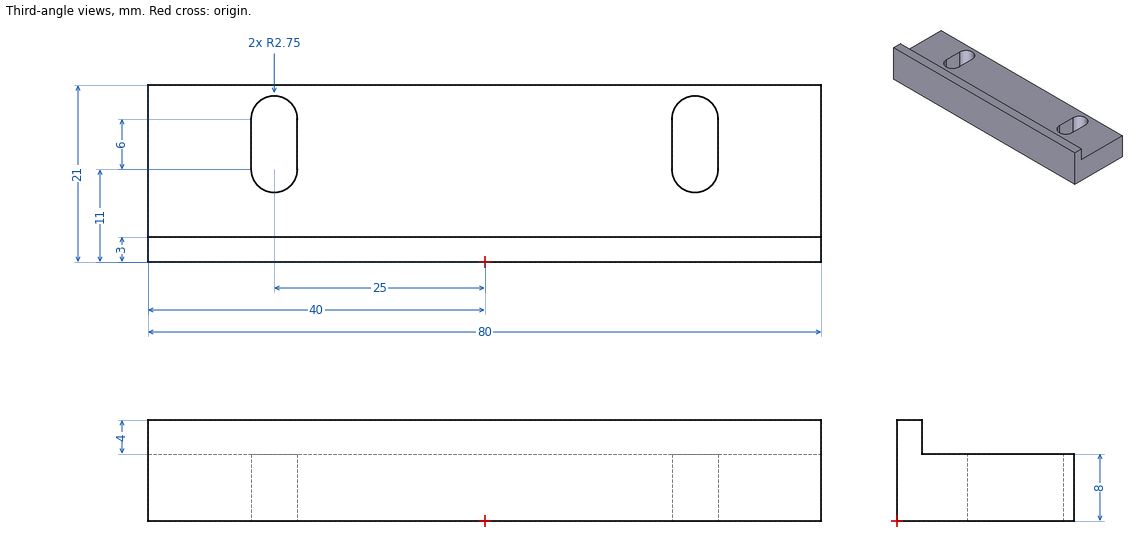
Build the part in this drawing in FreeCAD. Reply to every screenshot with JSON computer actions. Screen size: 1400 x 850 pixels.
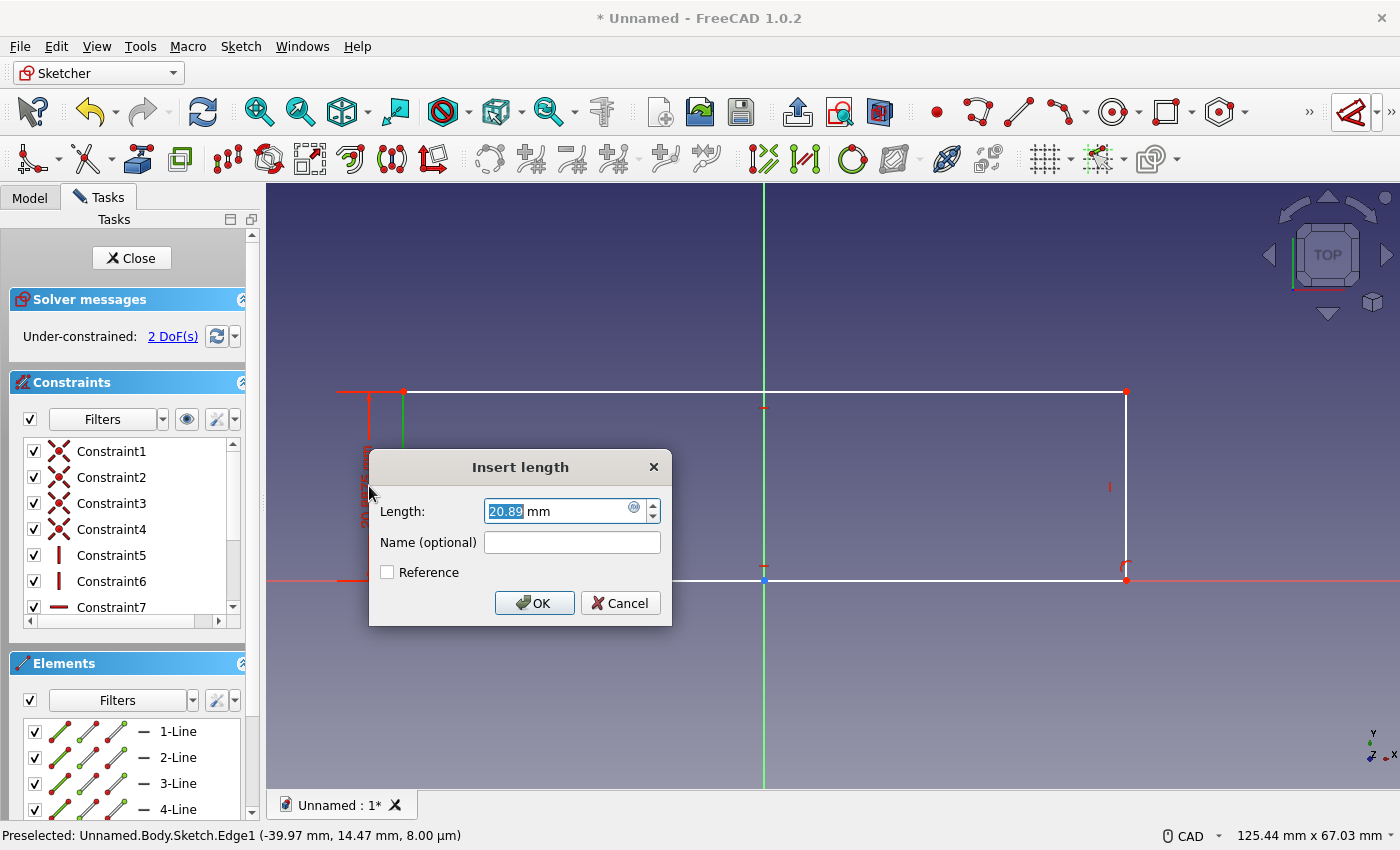
{"action": "type", "text": "21"}
{"action": "key", "text": "Return"}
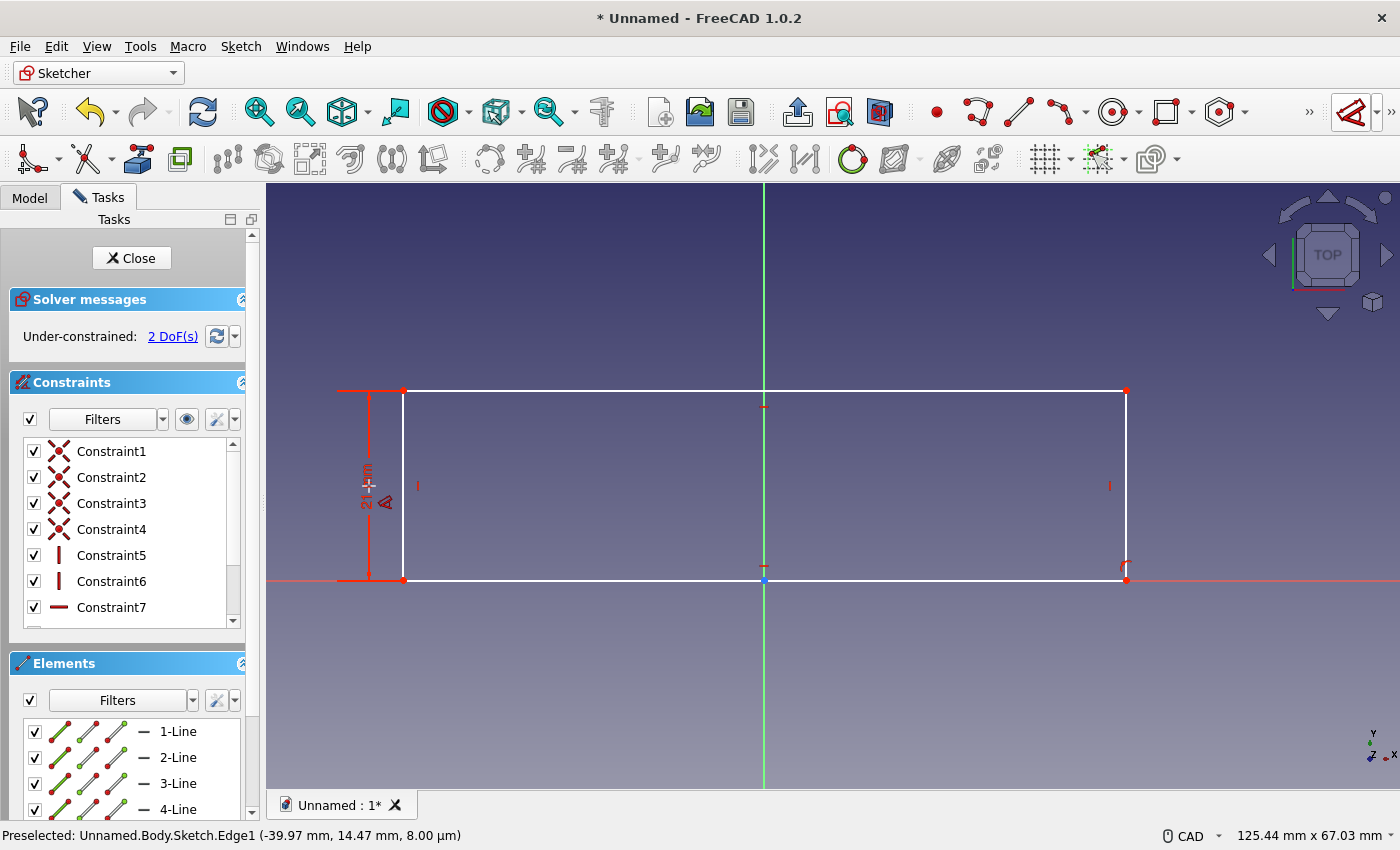
{"action": "left_click", "coordinate": [620, 581]}
{"action": "left_click", "coordinate": [598, 615]}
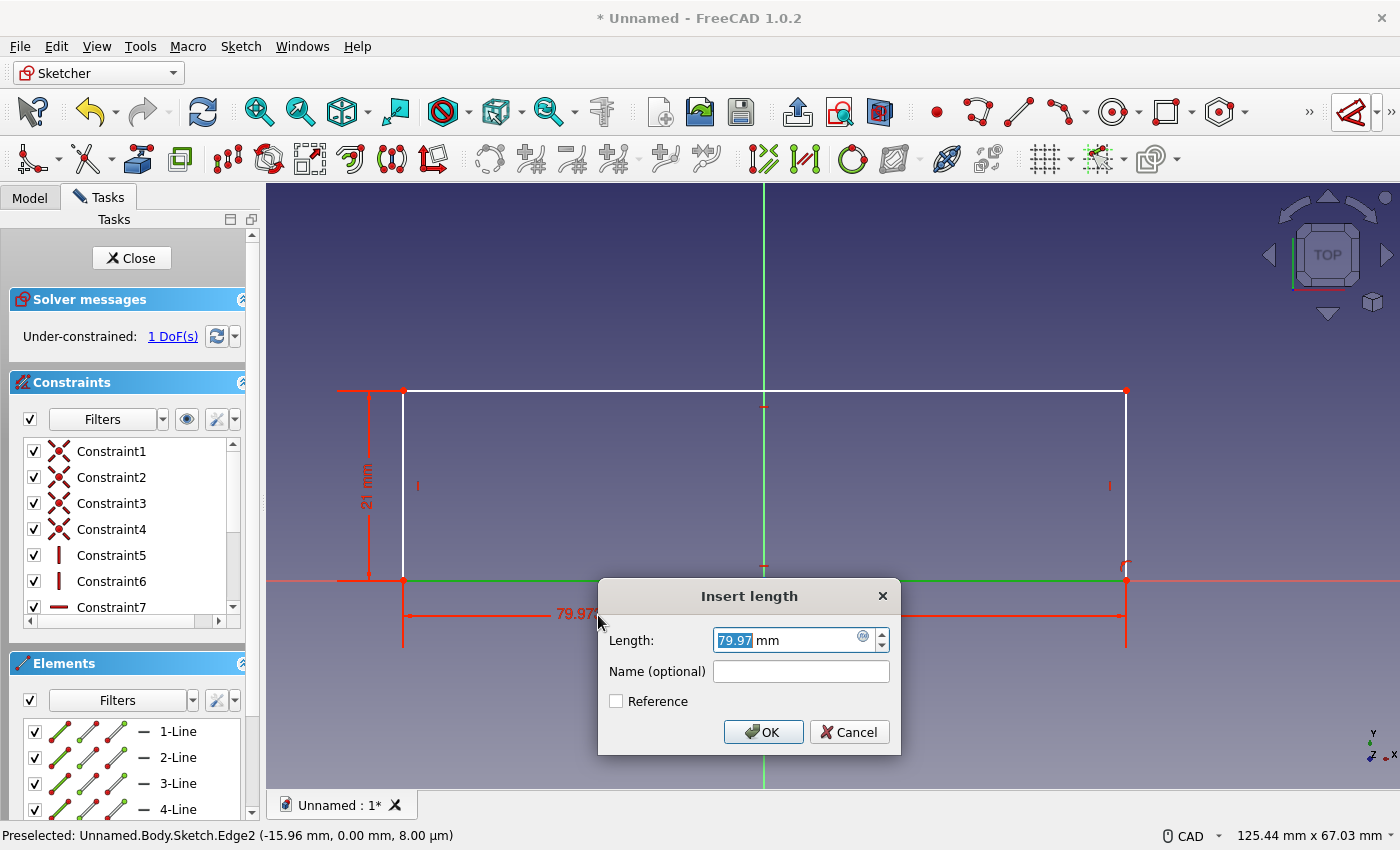
{"action": "type", "text": "80"}
{"action": "key", "text": "Return"}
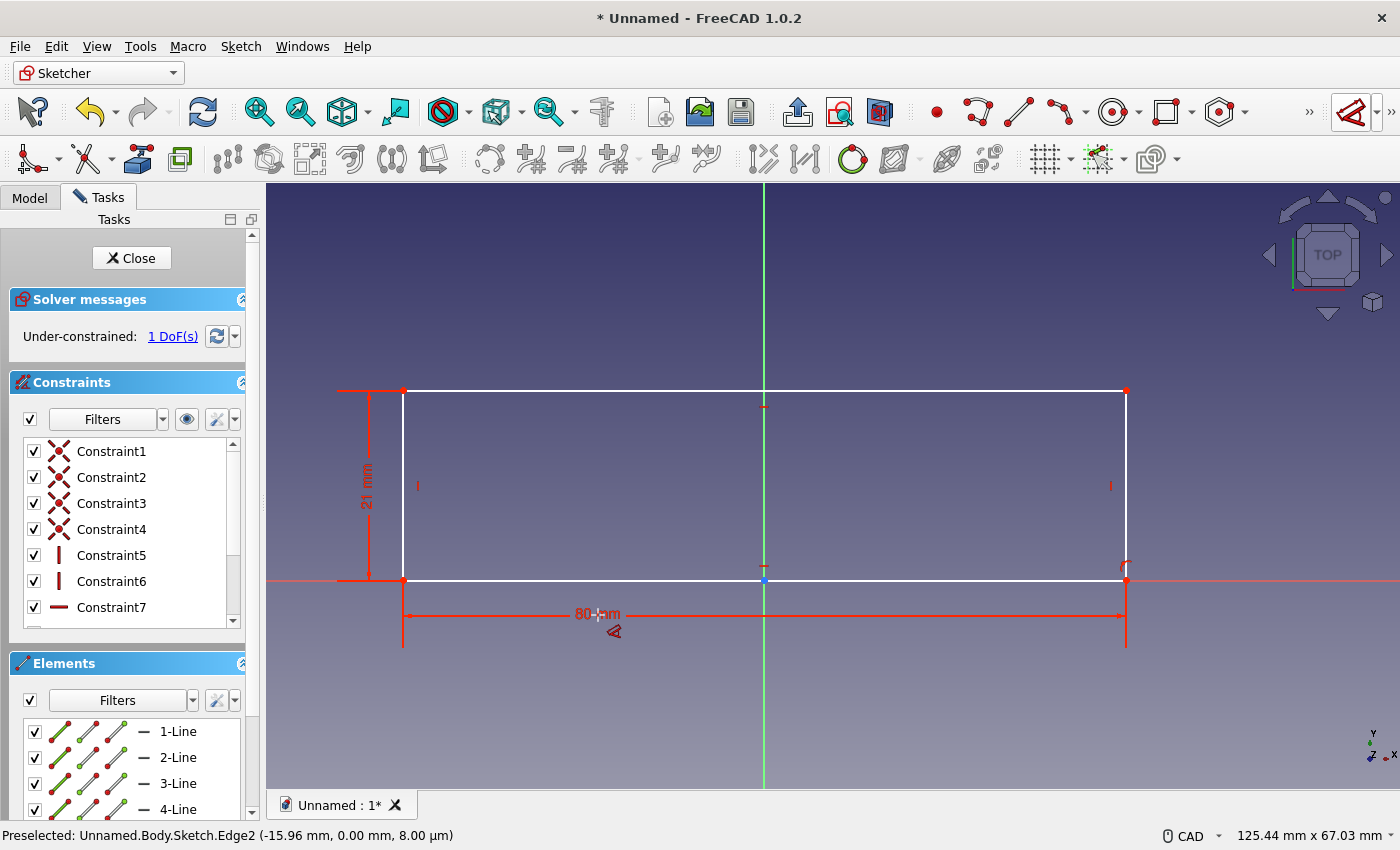
{"action": "left_click", "coordinate": [403, 391]}
{"action": "left_click", "coordinate": [501, 615]}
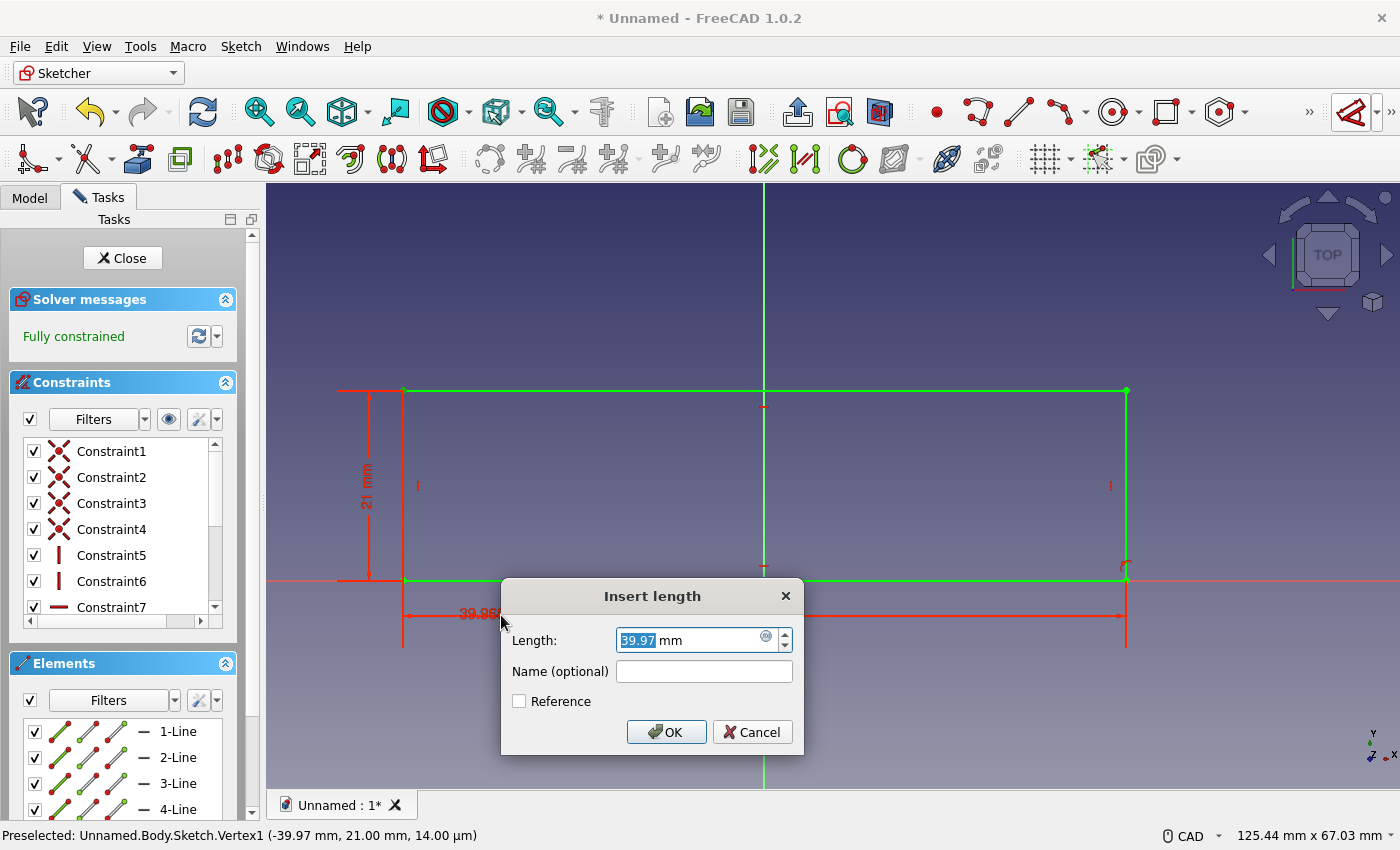
{"action": "type", "text": "40"}
{"action": "key", "text": "Return"}
{"action": "key", "text": "Escape"}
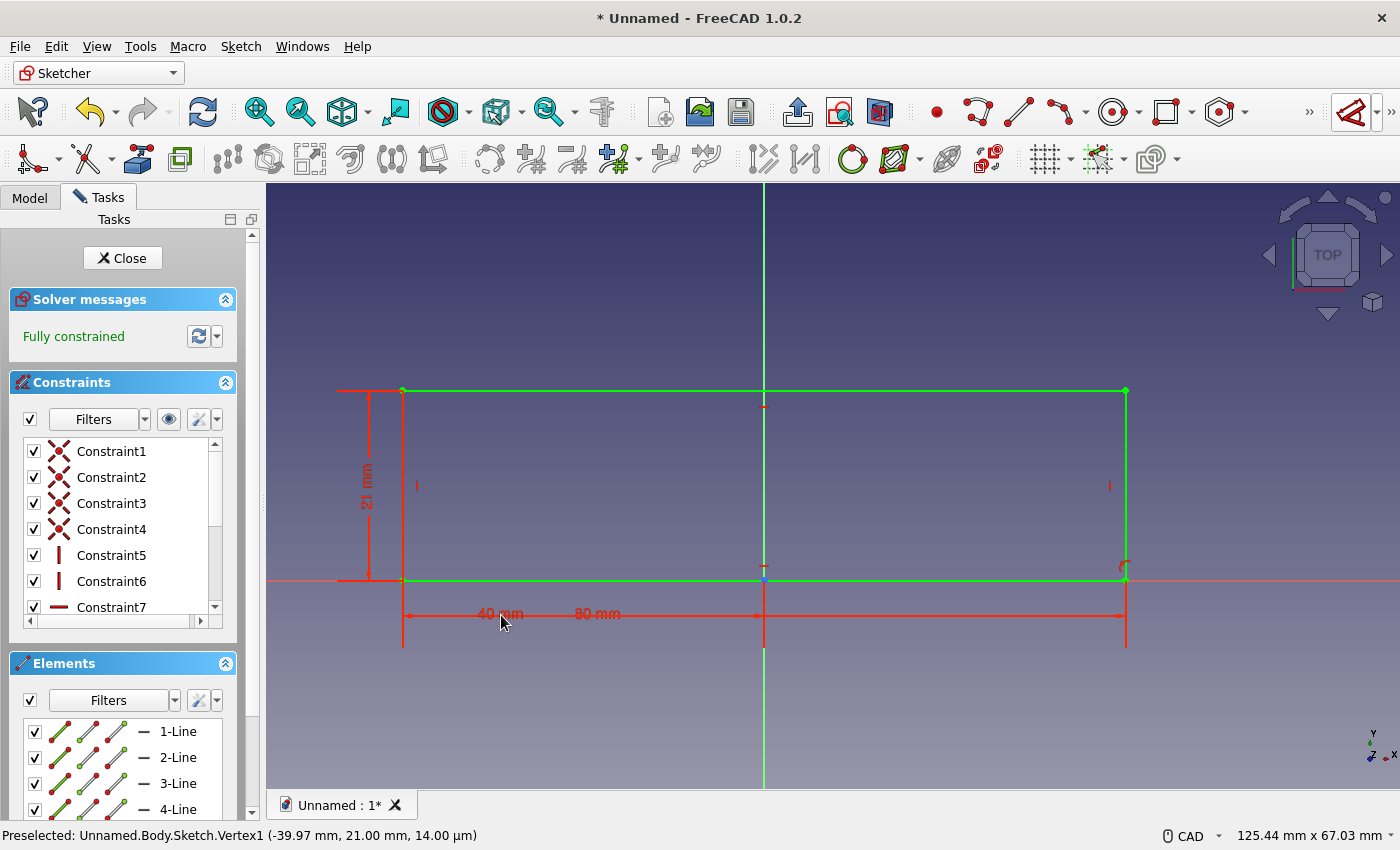
{"action": "left_click", "coordinate": [123, 258]}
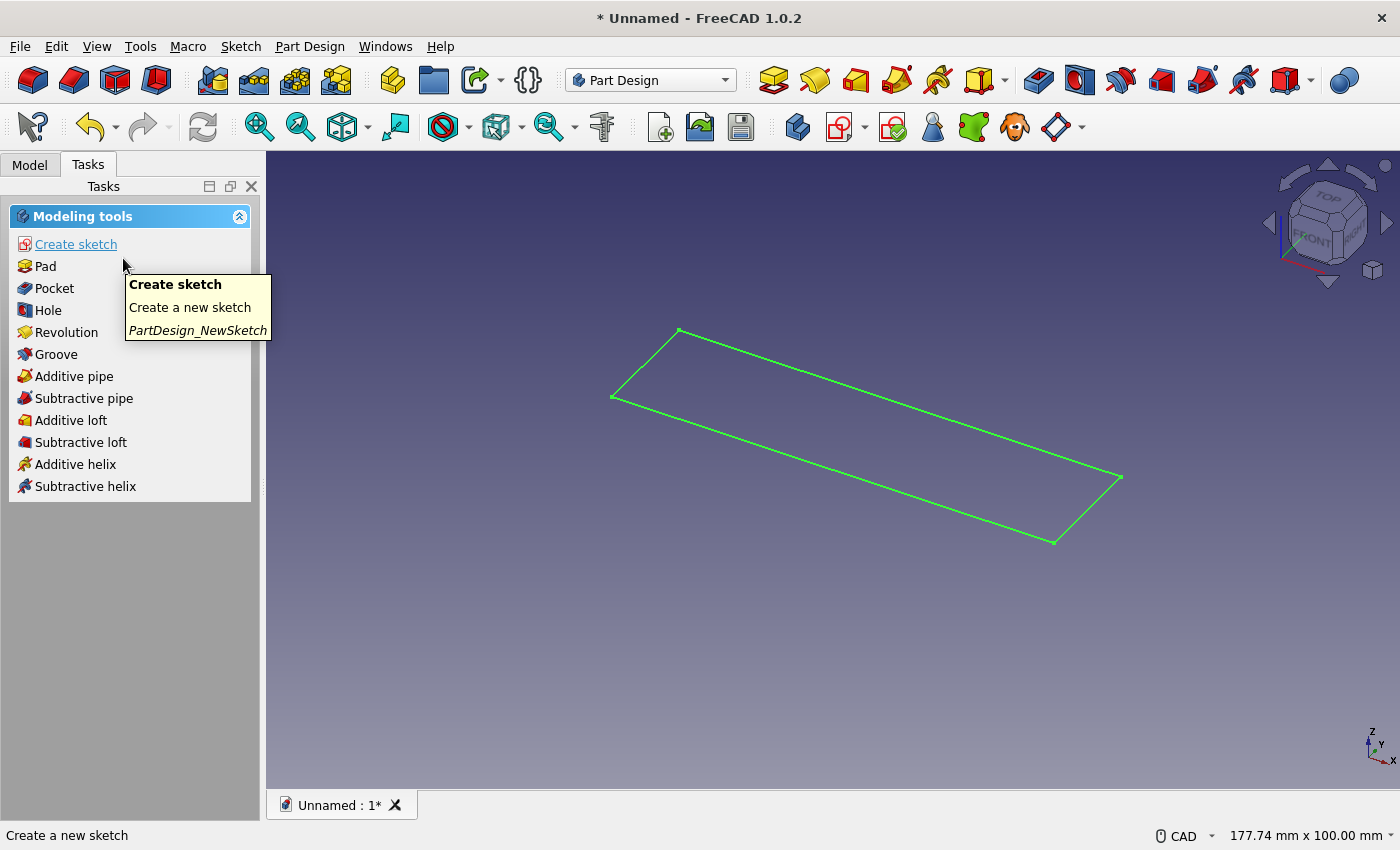
{"action": "left_click", "coordinate": [774, 80]}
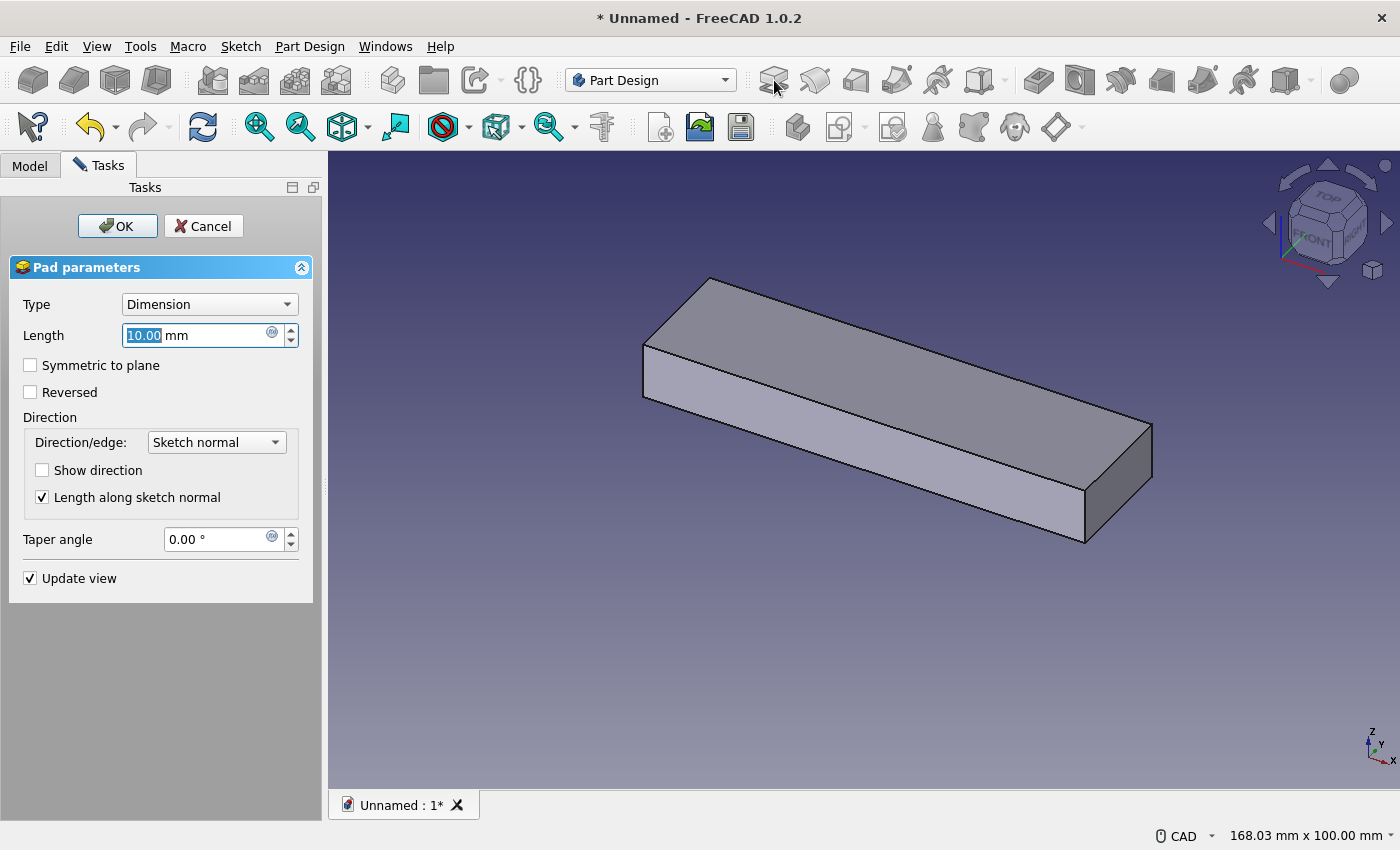
{"action": "type", "text": "8"}
{"action": "key", "text": "Tab"}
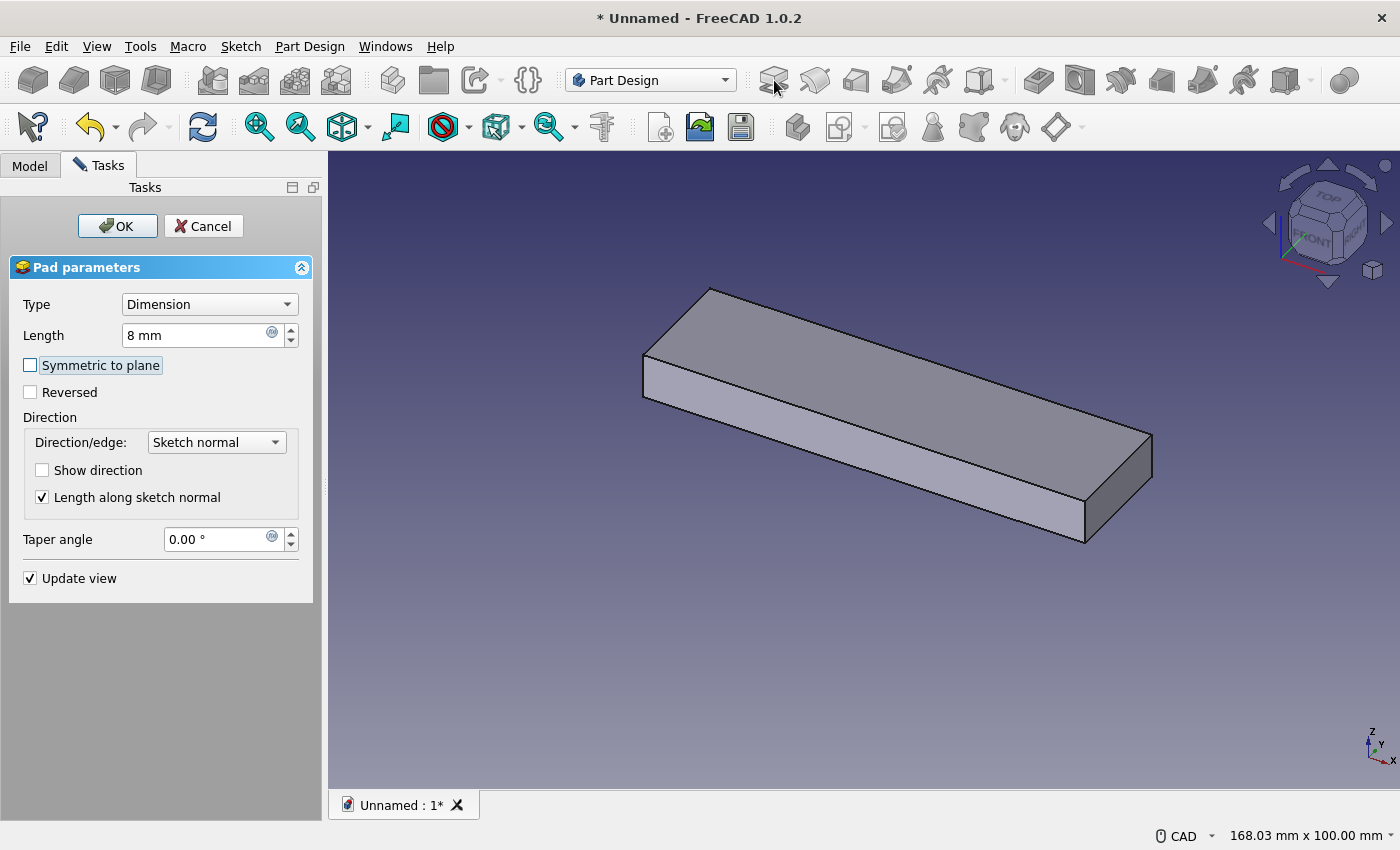
{"action": "left_click", "coordinate": [118, 226]}